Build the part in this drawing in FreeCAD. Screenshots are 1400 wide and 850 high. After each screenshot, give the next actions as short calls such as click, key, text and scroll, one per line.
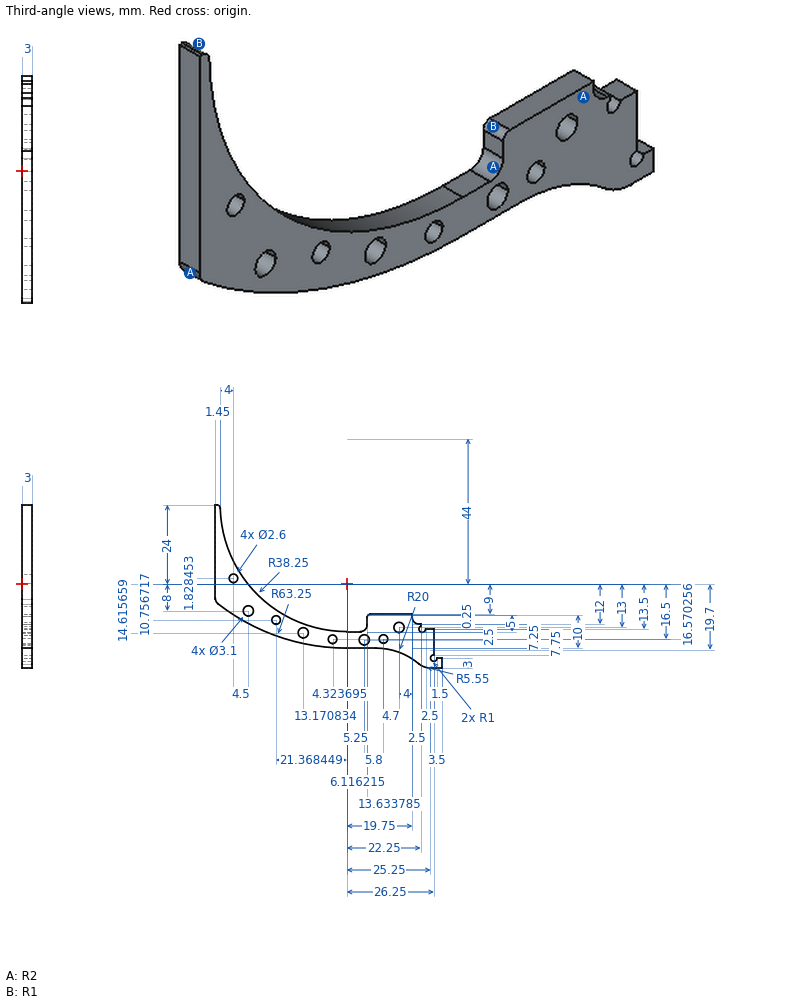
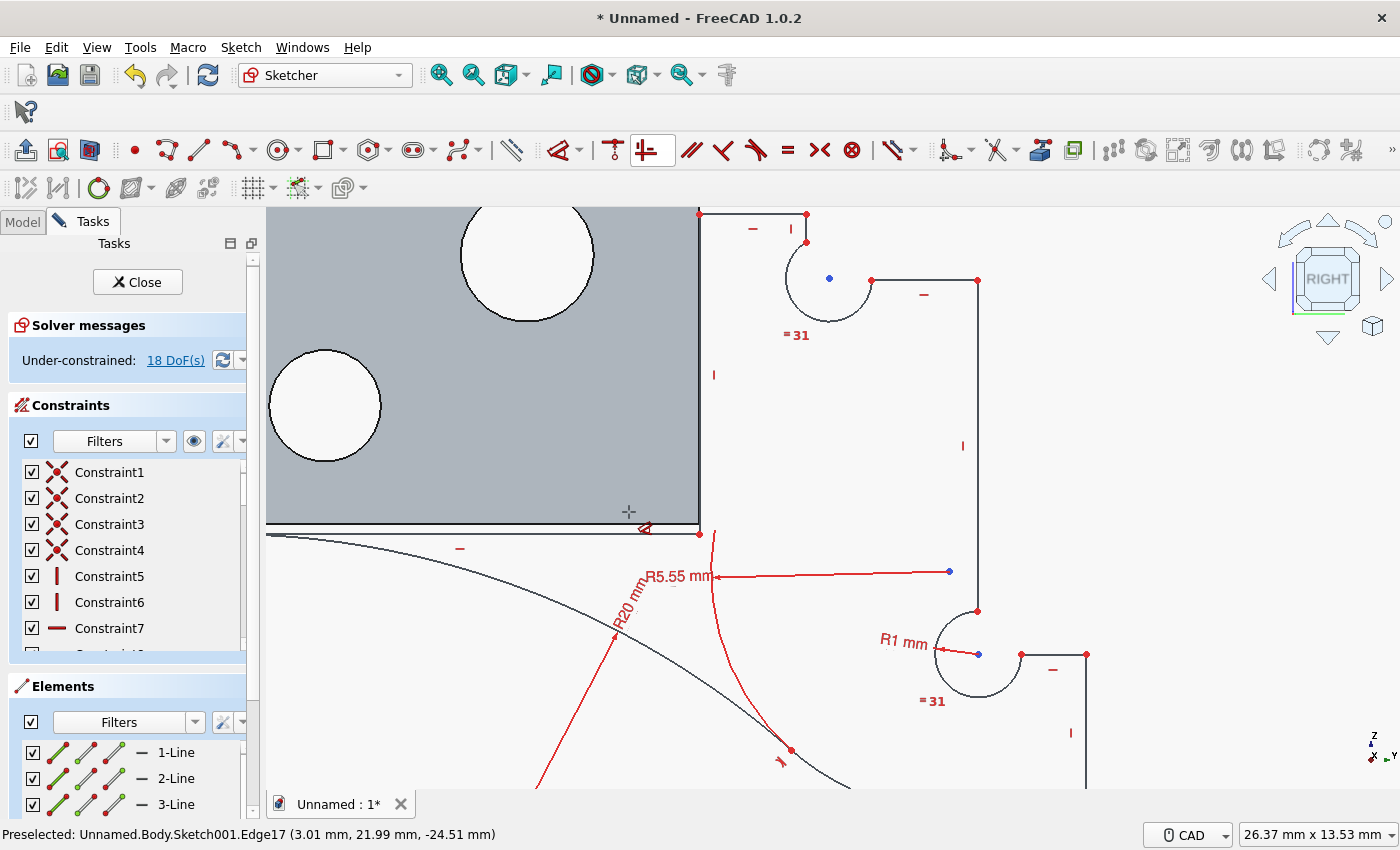
click(1086, 702)
click(1120, 708)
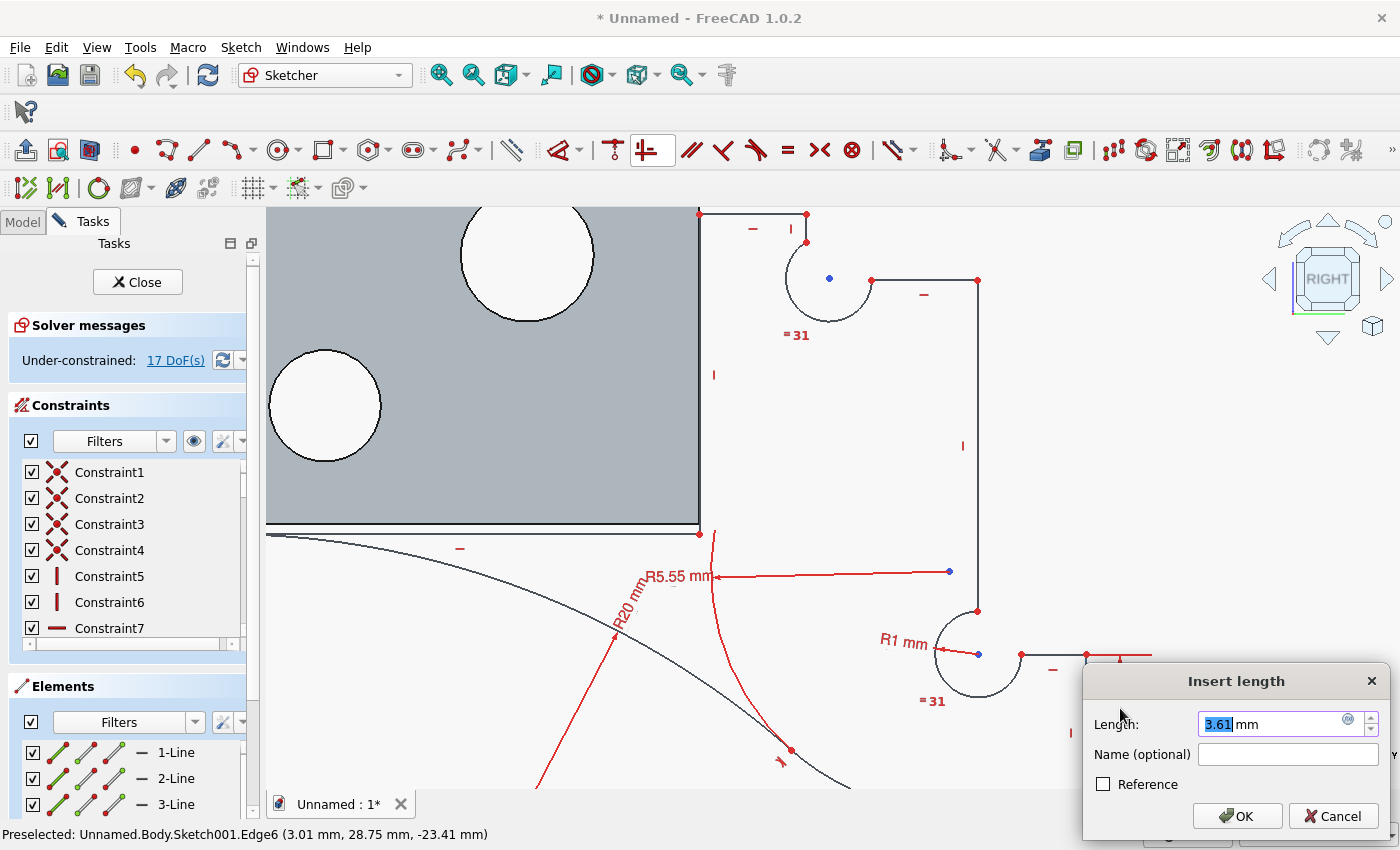
text(3)
key(Return)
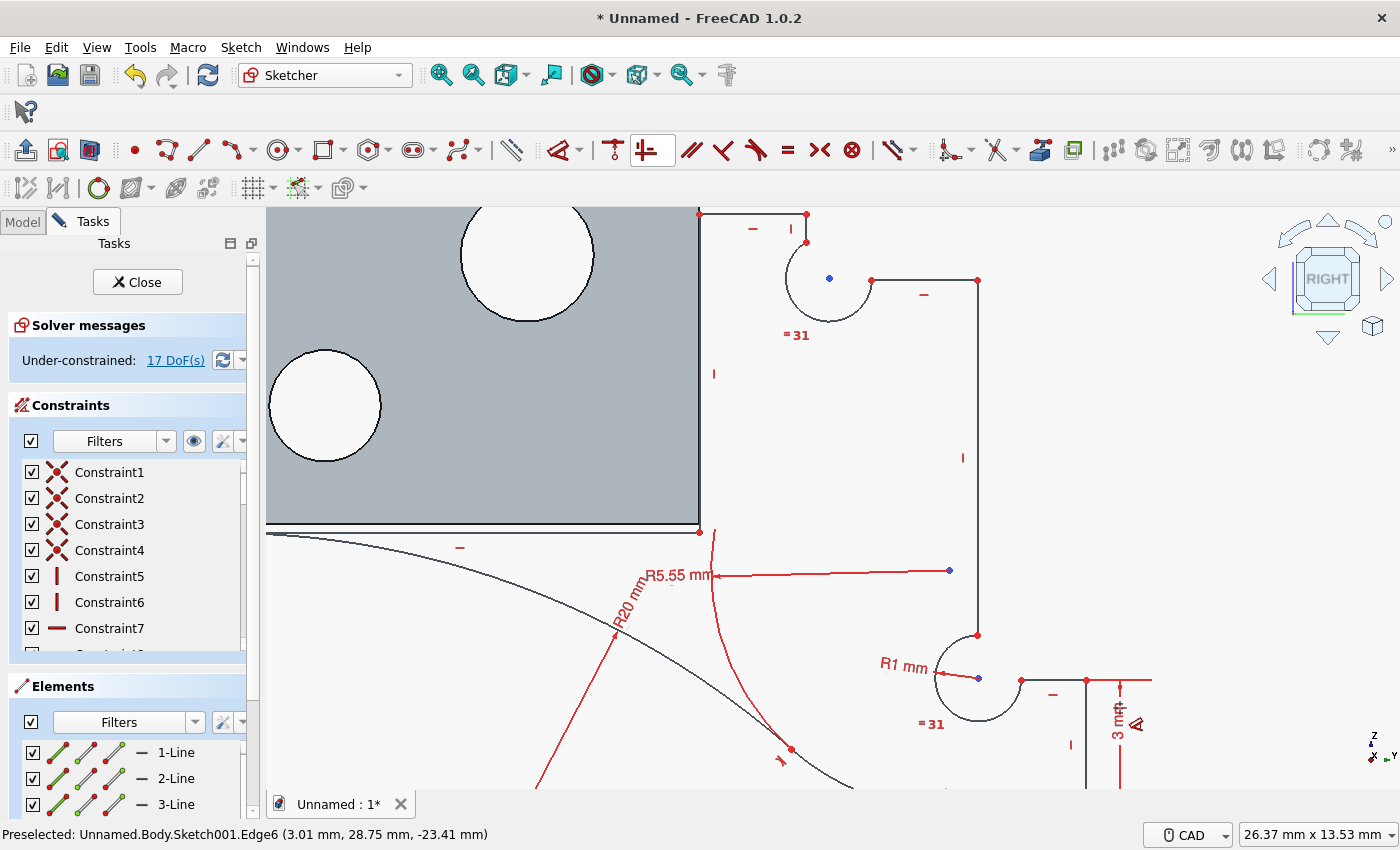
scroll(937, 649, down, 5)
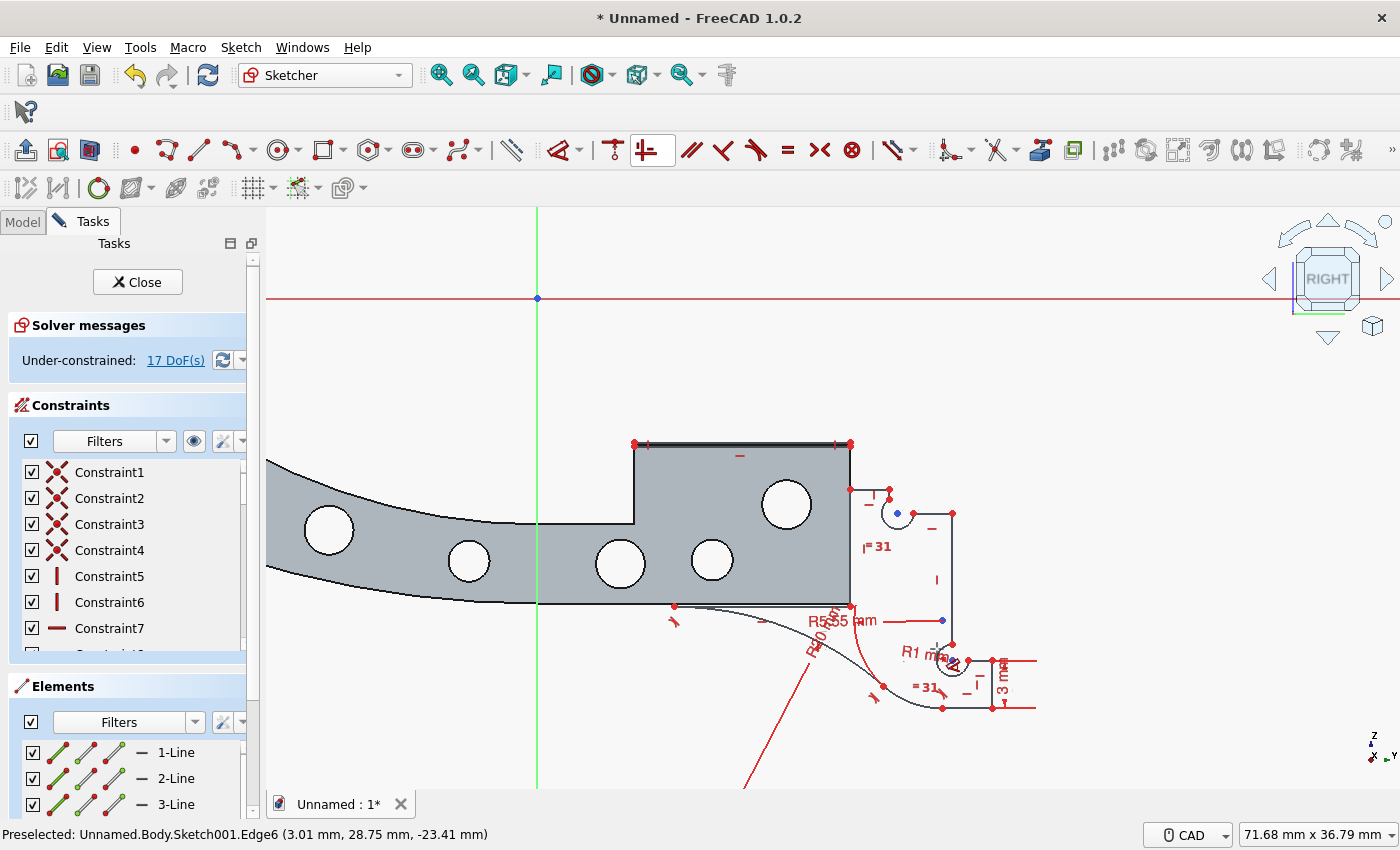
scroll(634, 443, up, 6)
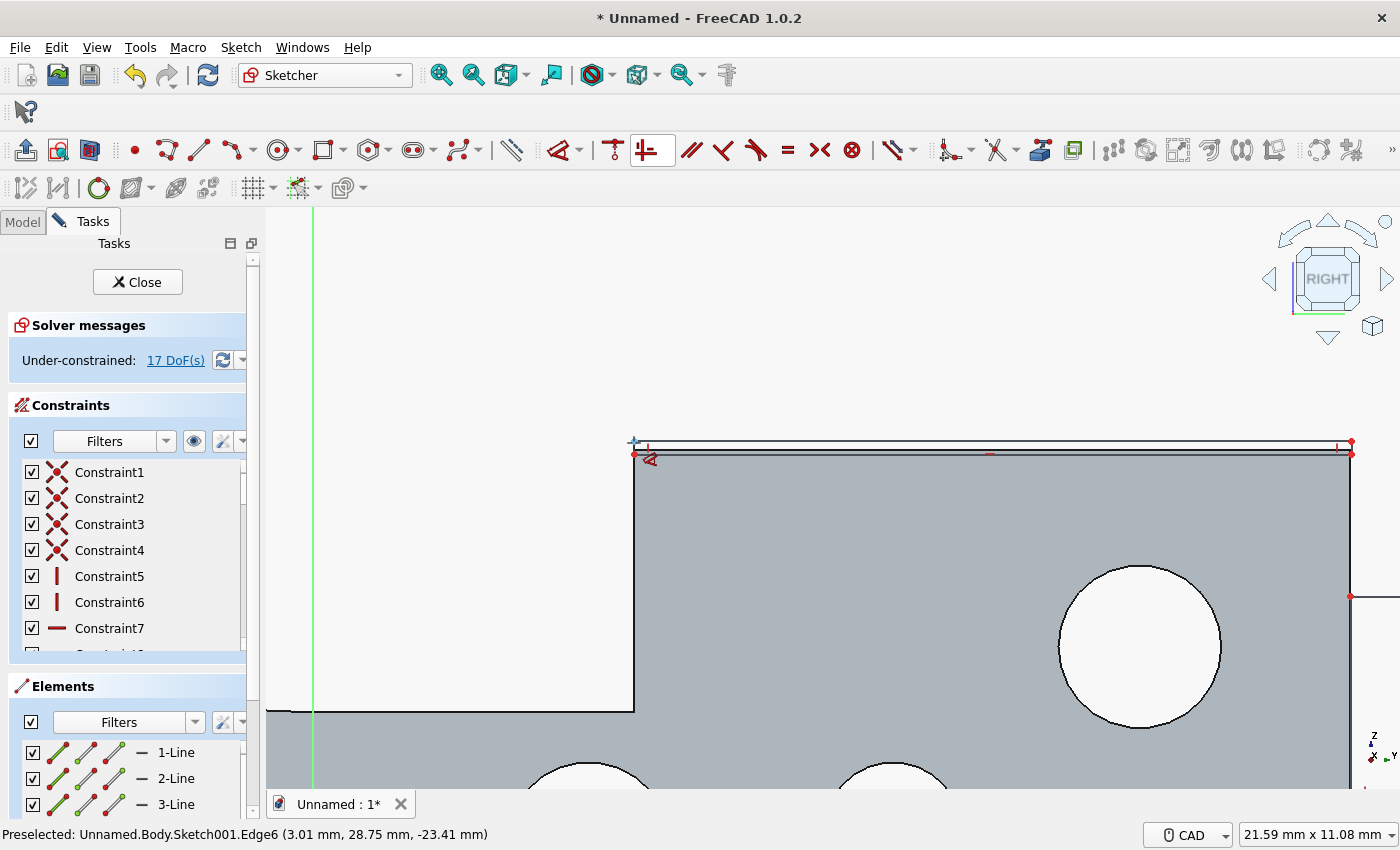
click(634, 441)
click(668, 338)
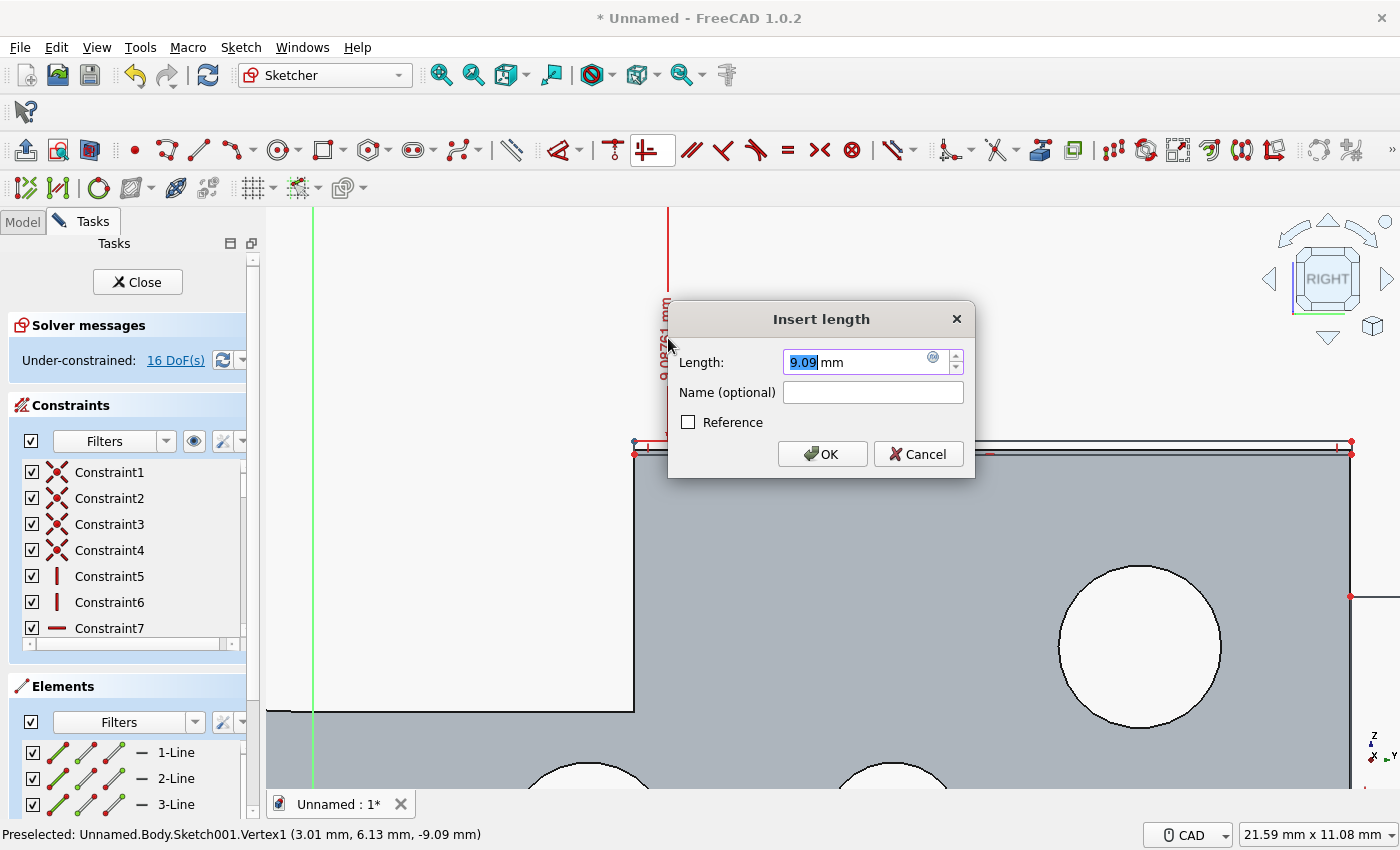
text(9)
key(Return)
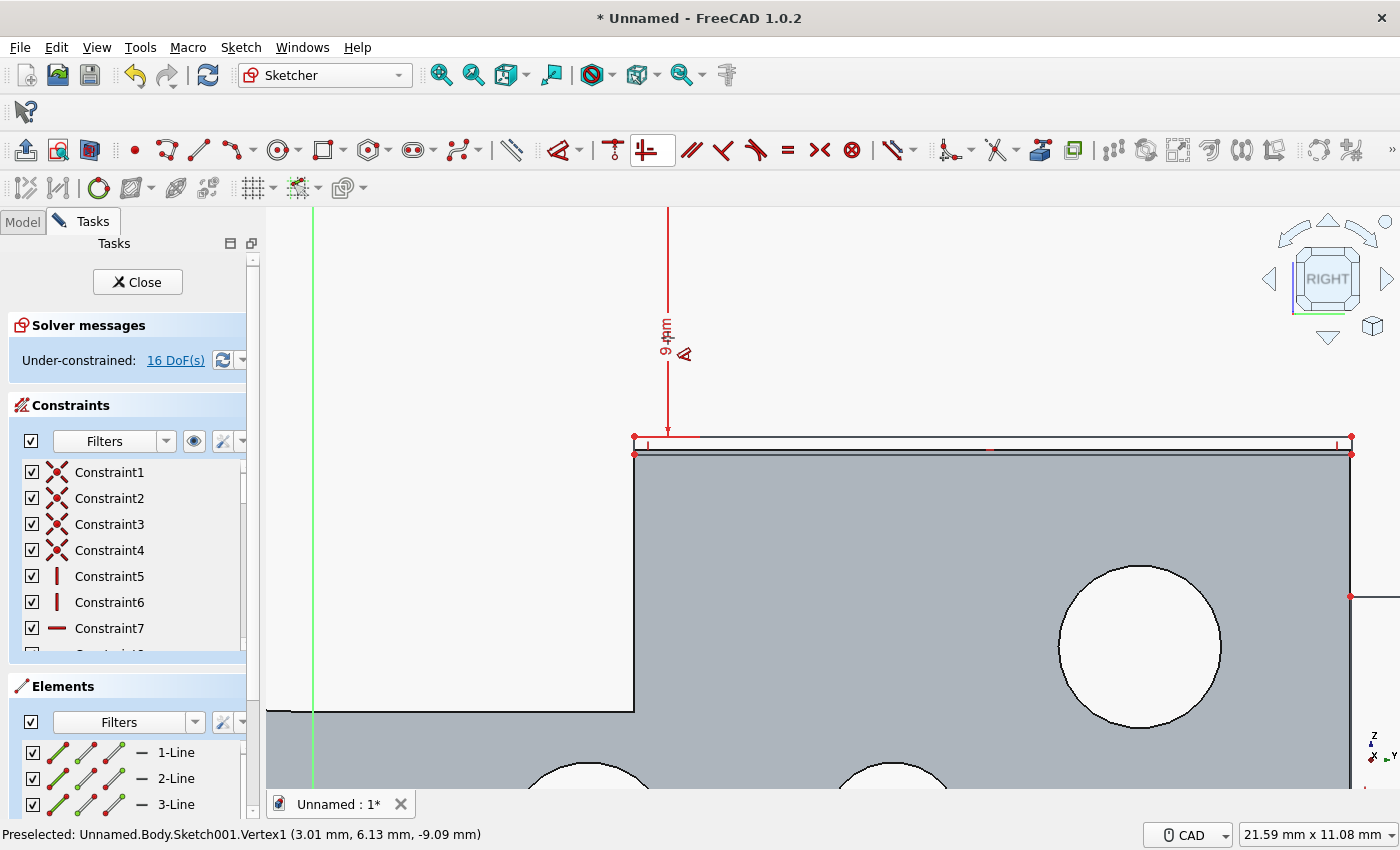
scroll(634, 442, down, 6)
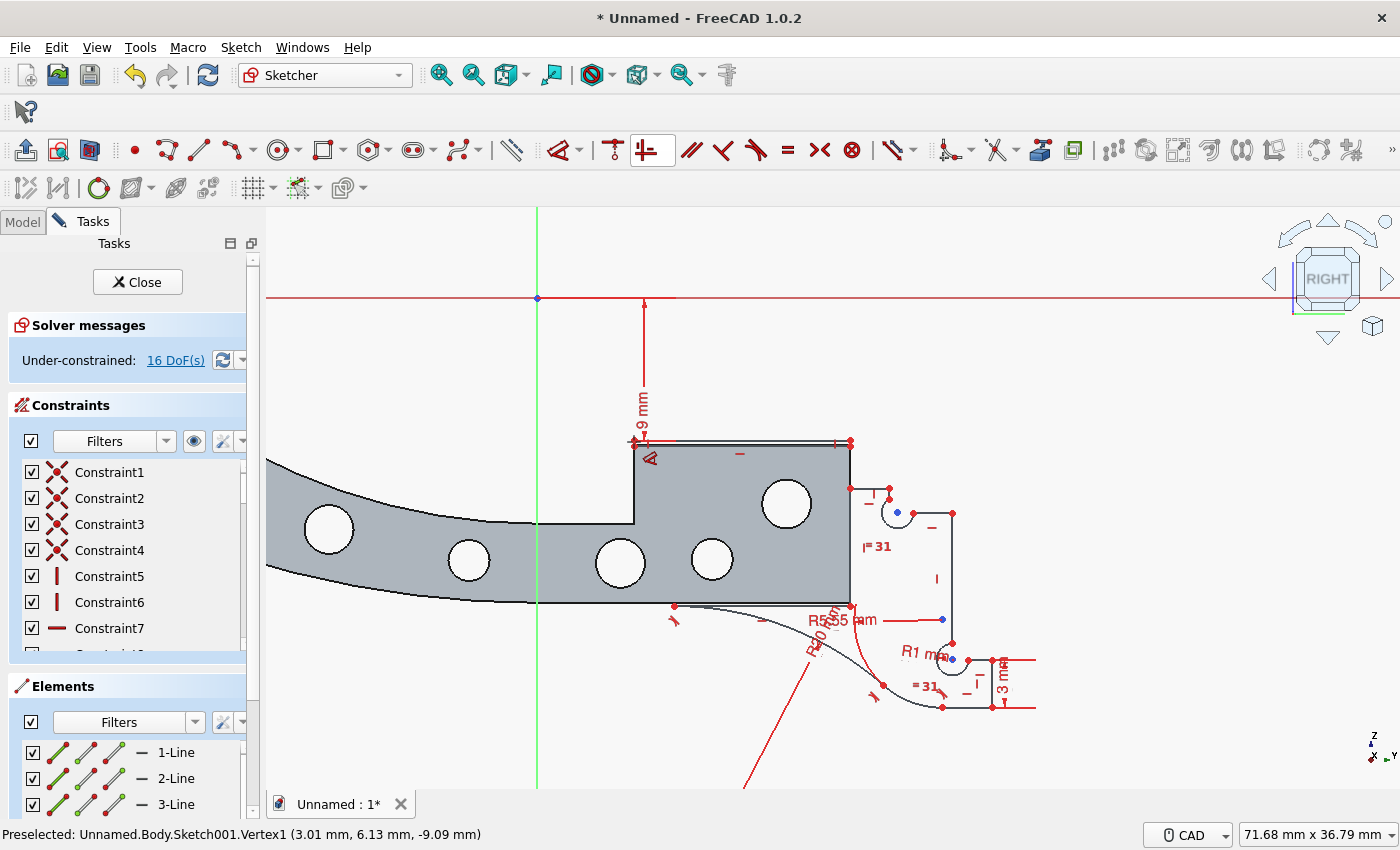
click(957, 708)
click(967, 742)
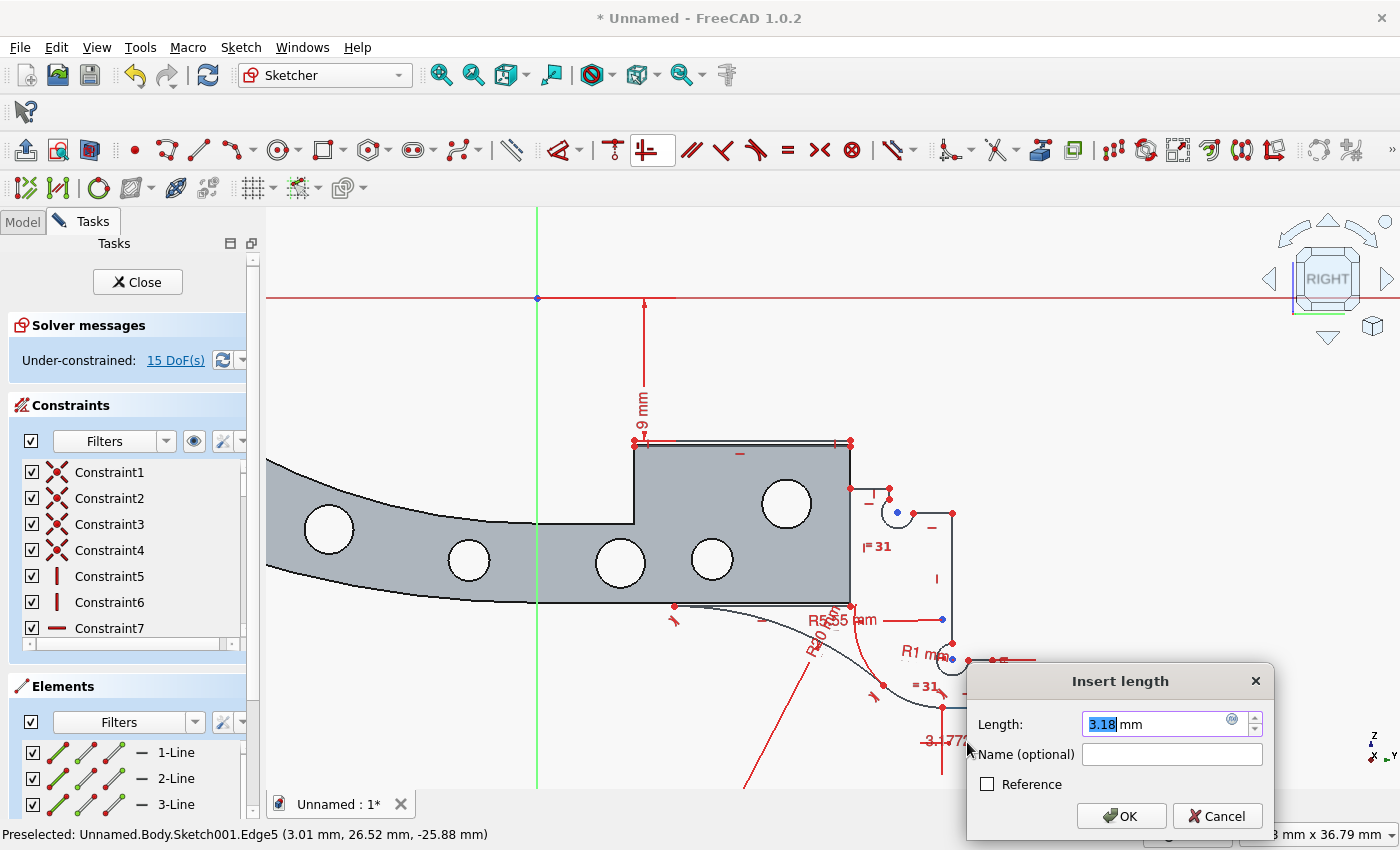
text(3.5)
key(Return)